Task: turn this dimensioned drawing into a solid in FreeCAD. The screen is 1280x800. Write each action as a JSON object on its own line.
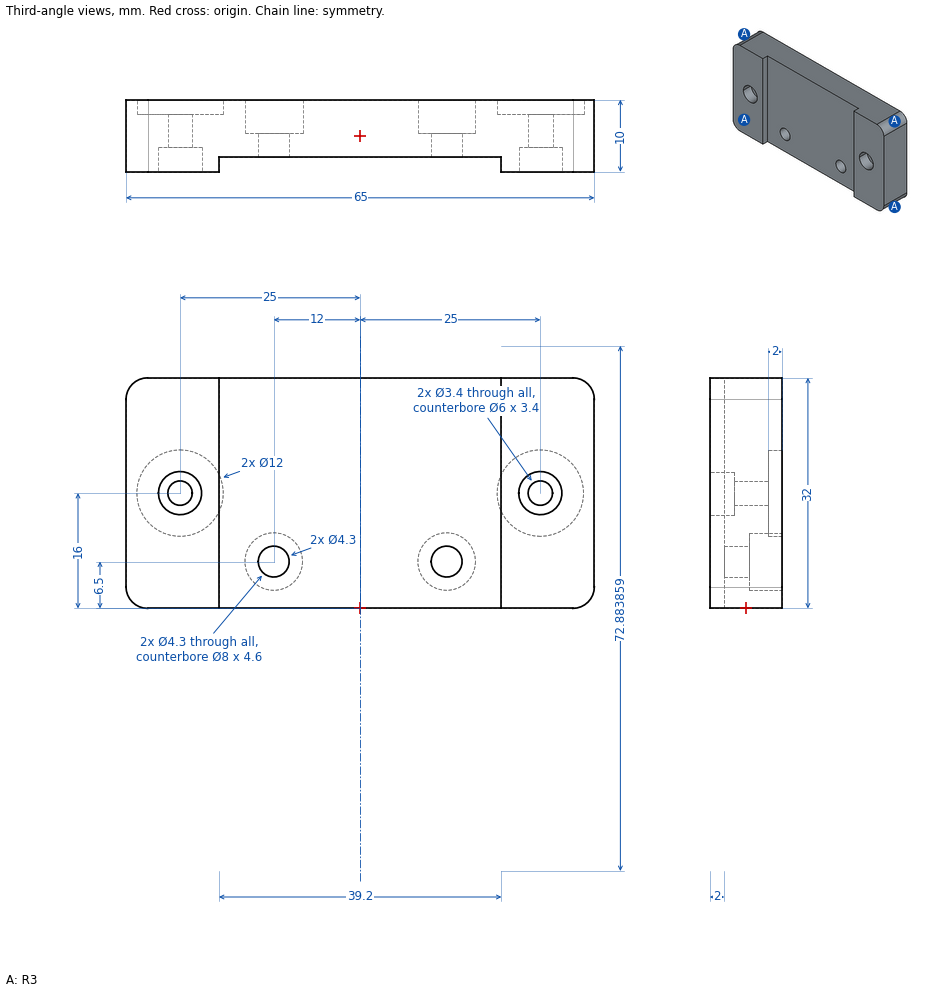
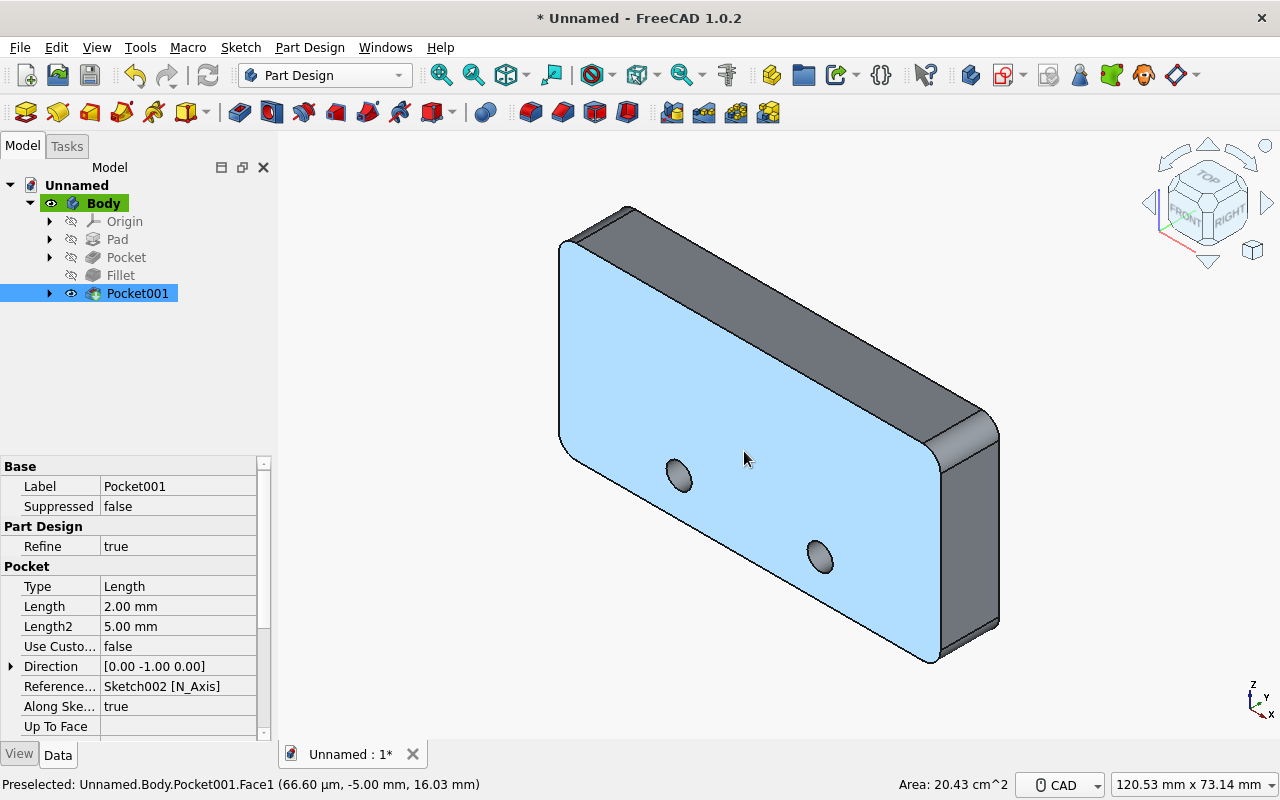
{"action": "left_click", "coordinate": [1004, 76]}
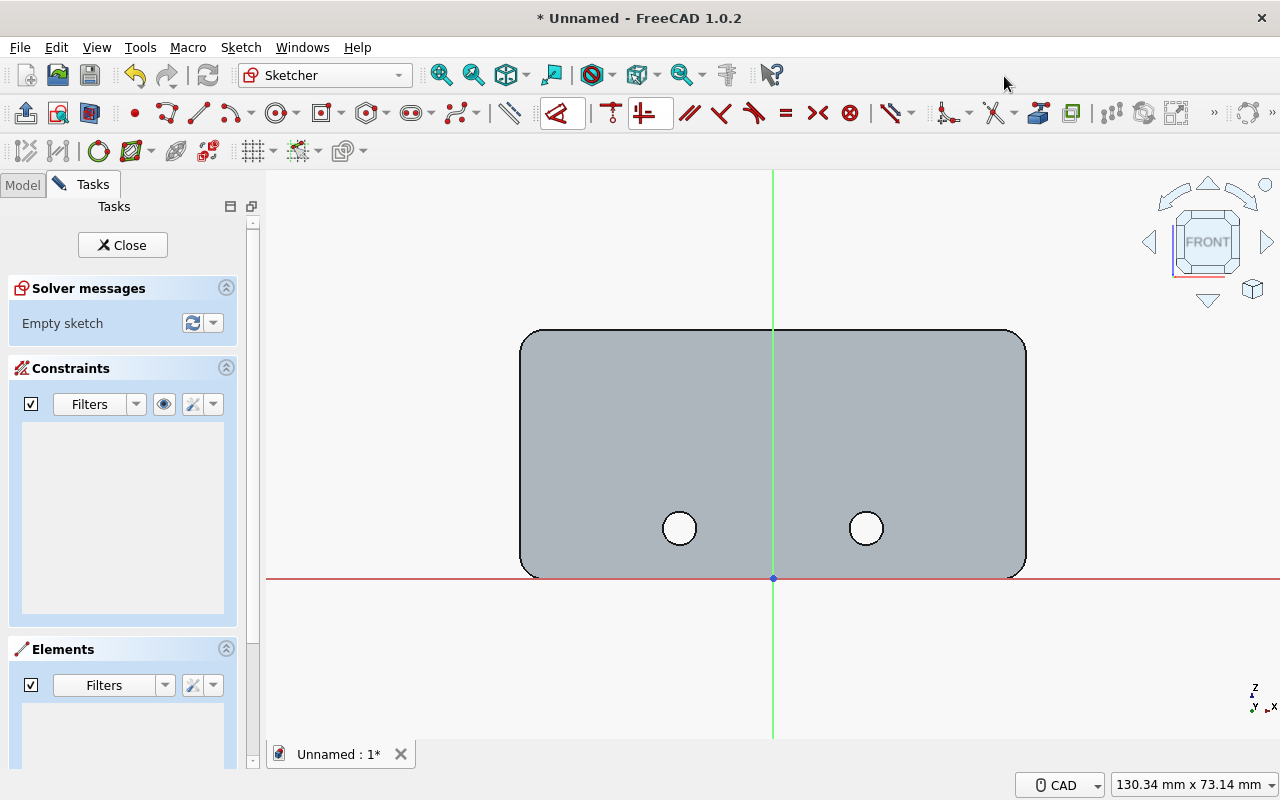
{"action": "scroll", "coordinate": [912, 623], "scroll_direction": "up", "scroll_amount": 2}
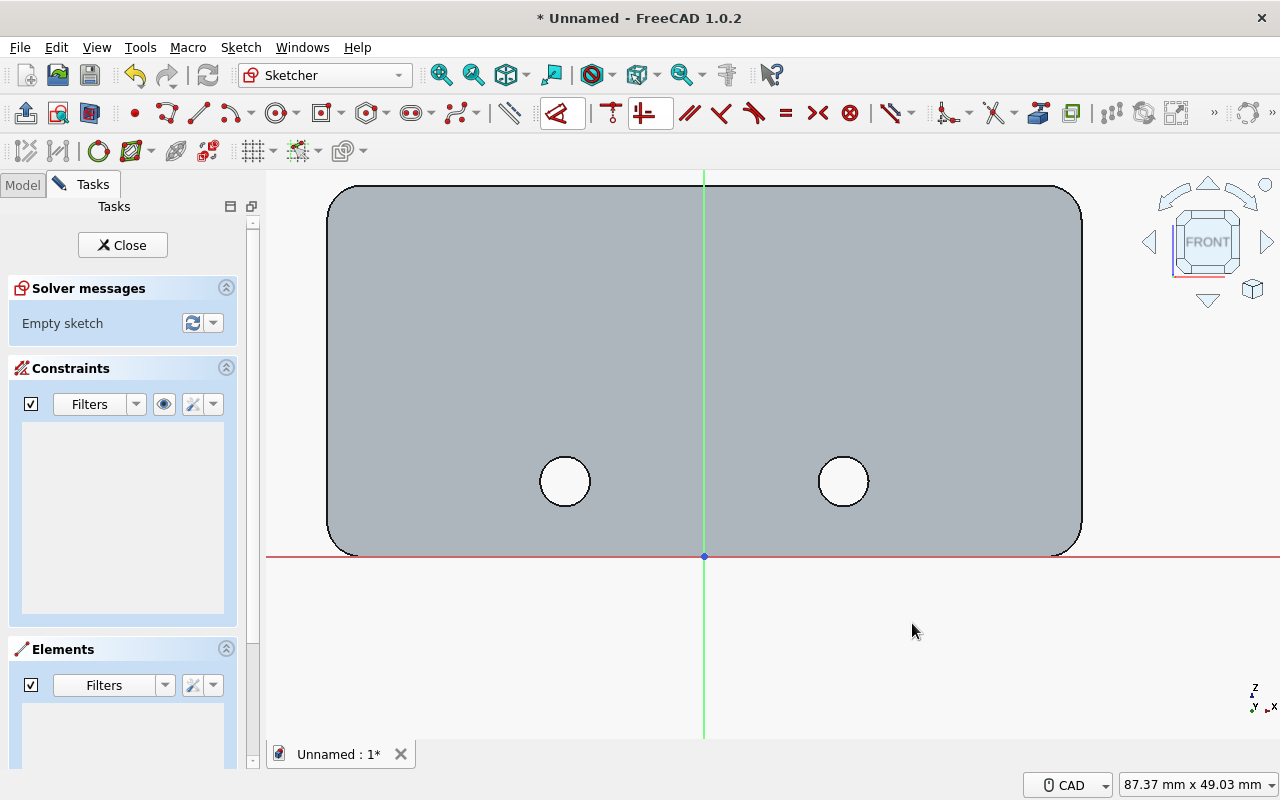
{"action": "left_click", "coordinate": [276, 114]}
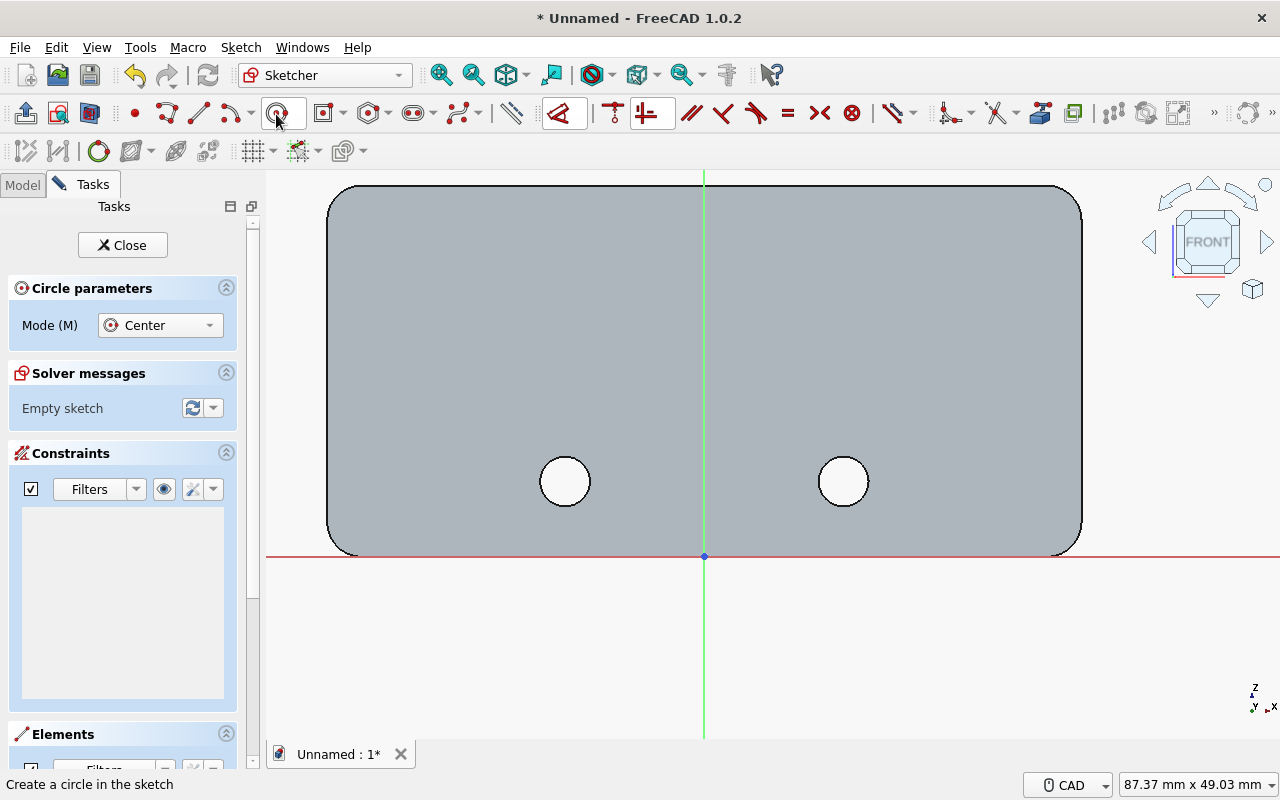
{"action": "left_click", "coordinate": [994, 371]}
{"action": "left_click", "coordinate": [1008, 357]}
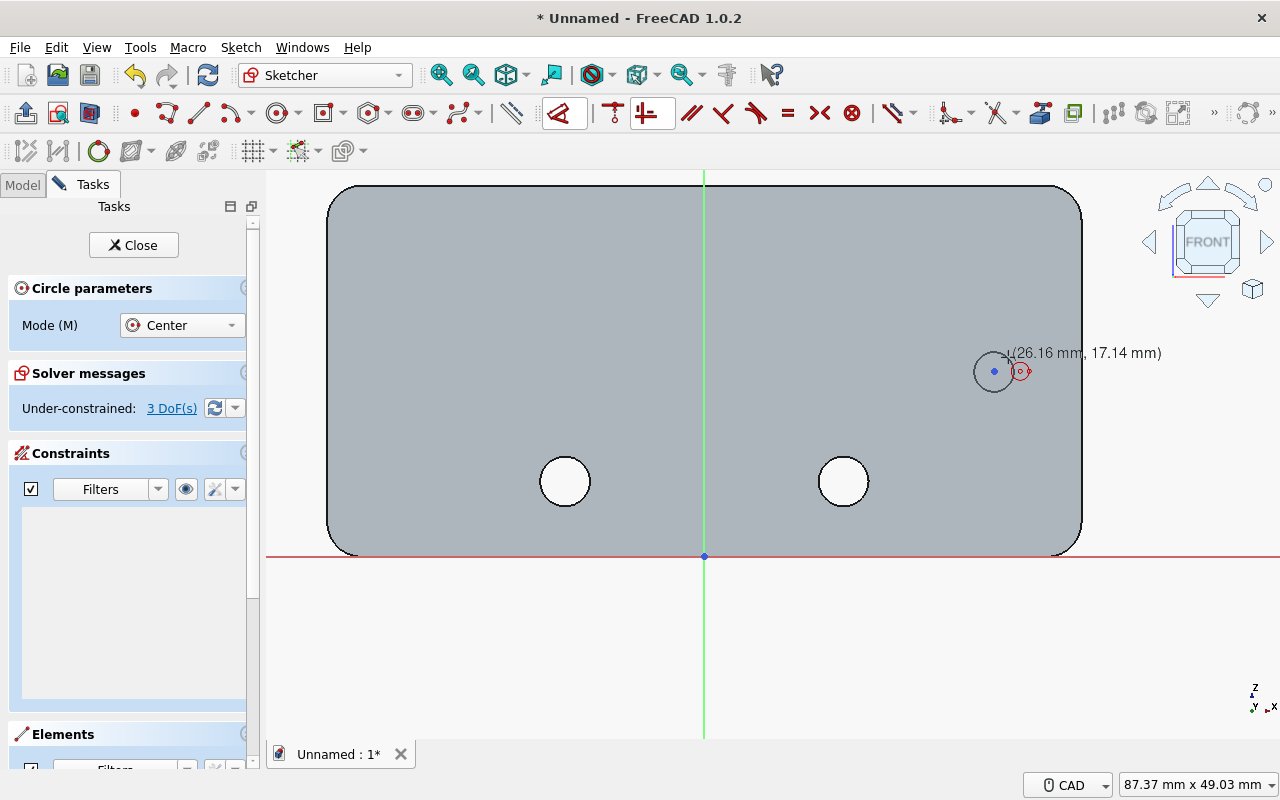
{"action": "left_click", "coordinate": [414, 371]}
{"action": "left_click", "coordinate": [428, 357]}
{"action": "key", "text": "Escape"}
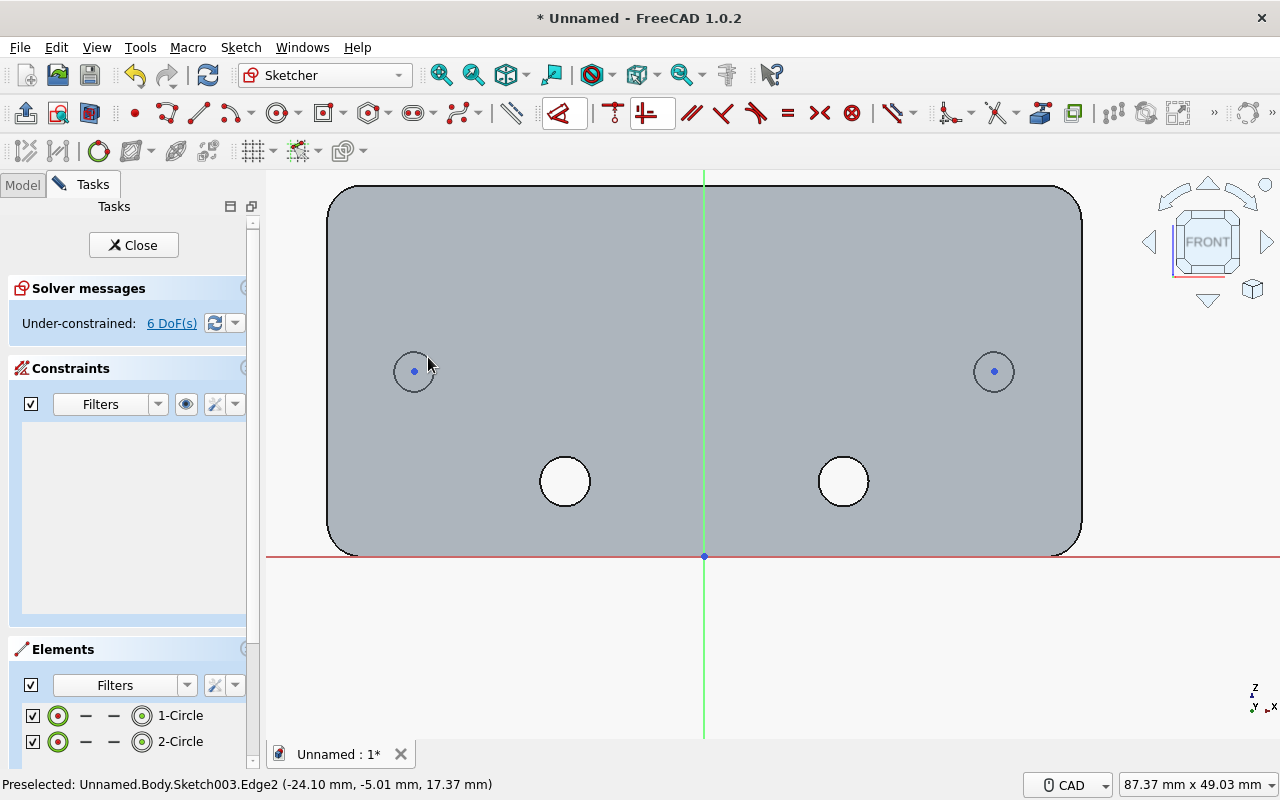
{"action": "left_click", "coordinate": [1008, 358]}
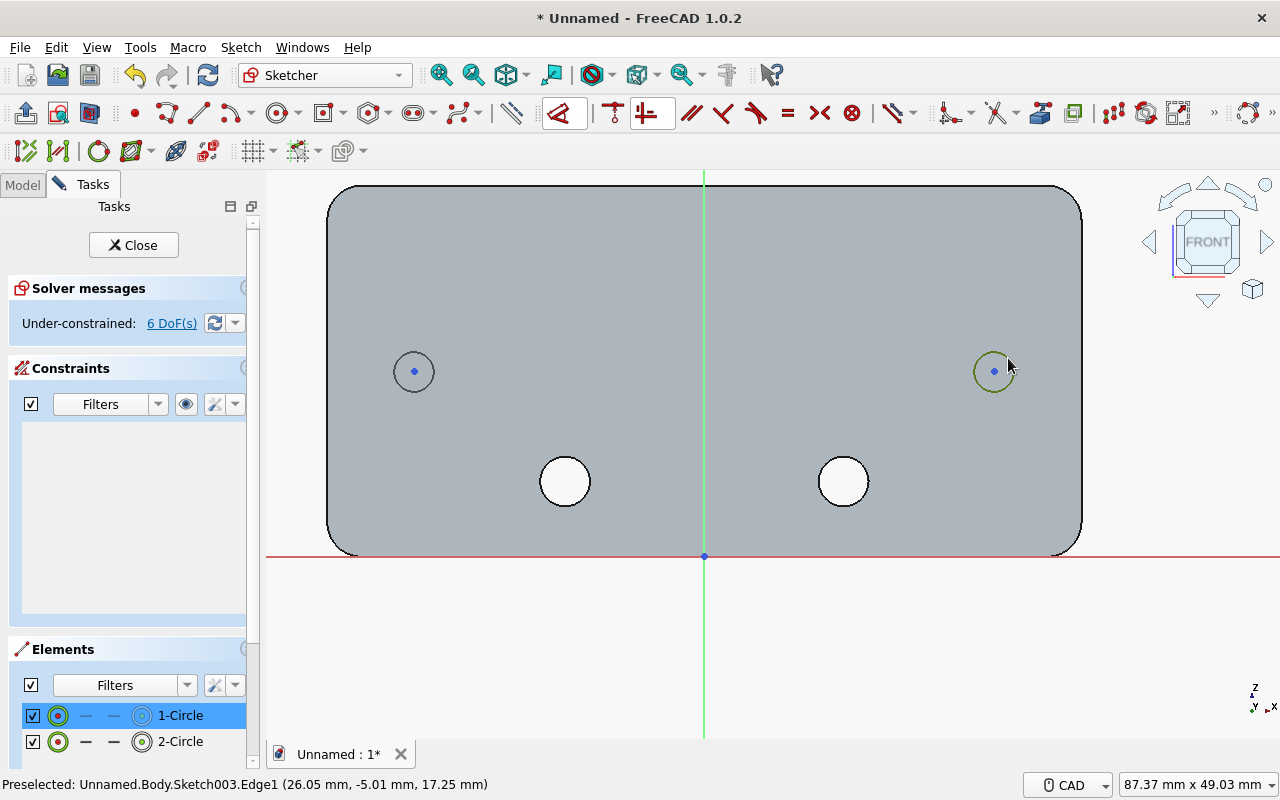
{"action": "left_click", "coordinate": [428, 358]}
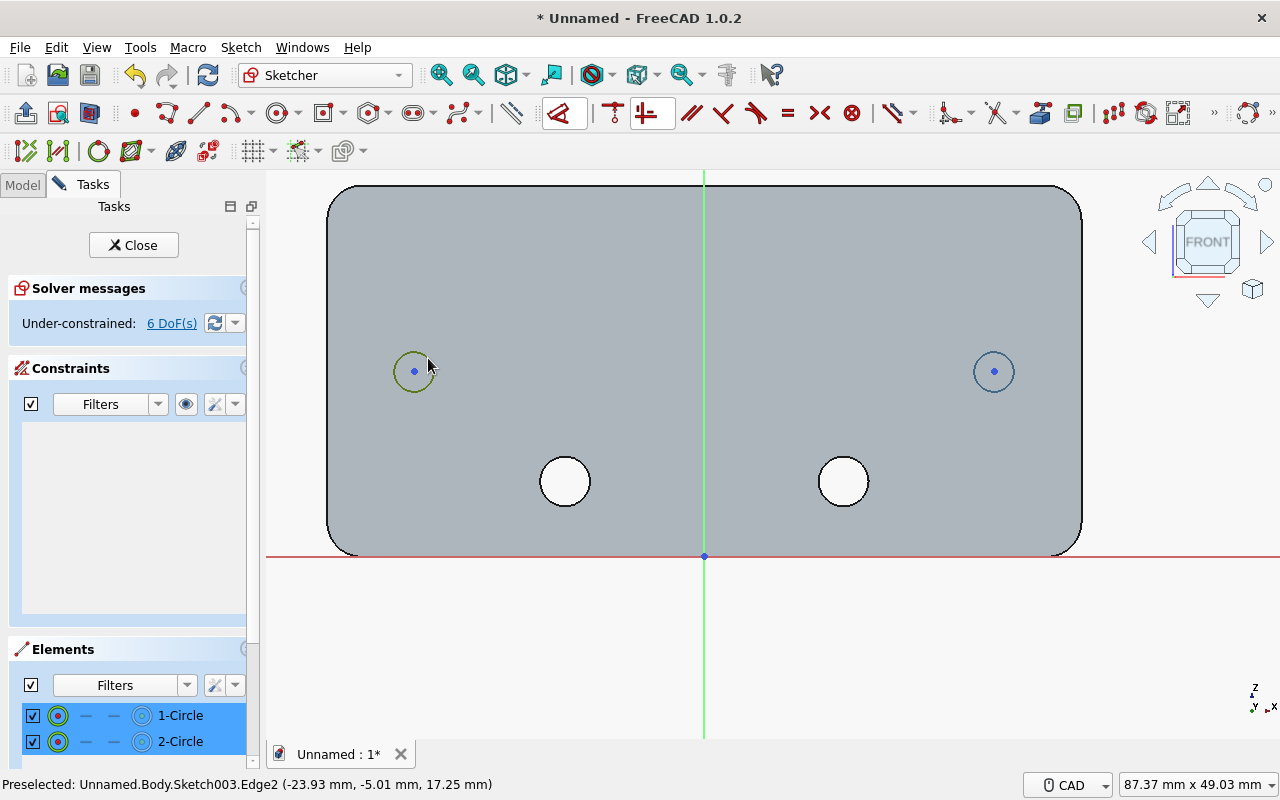
{"action": "left_click", "coordinate": [788, 114]}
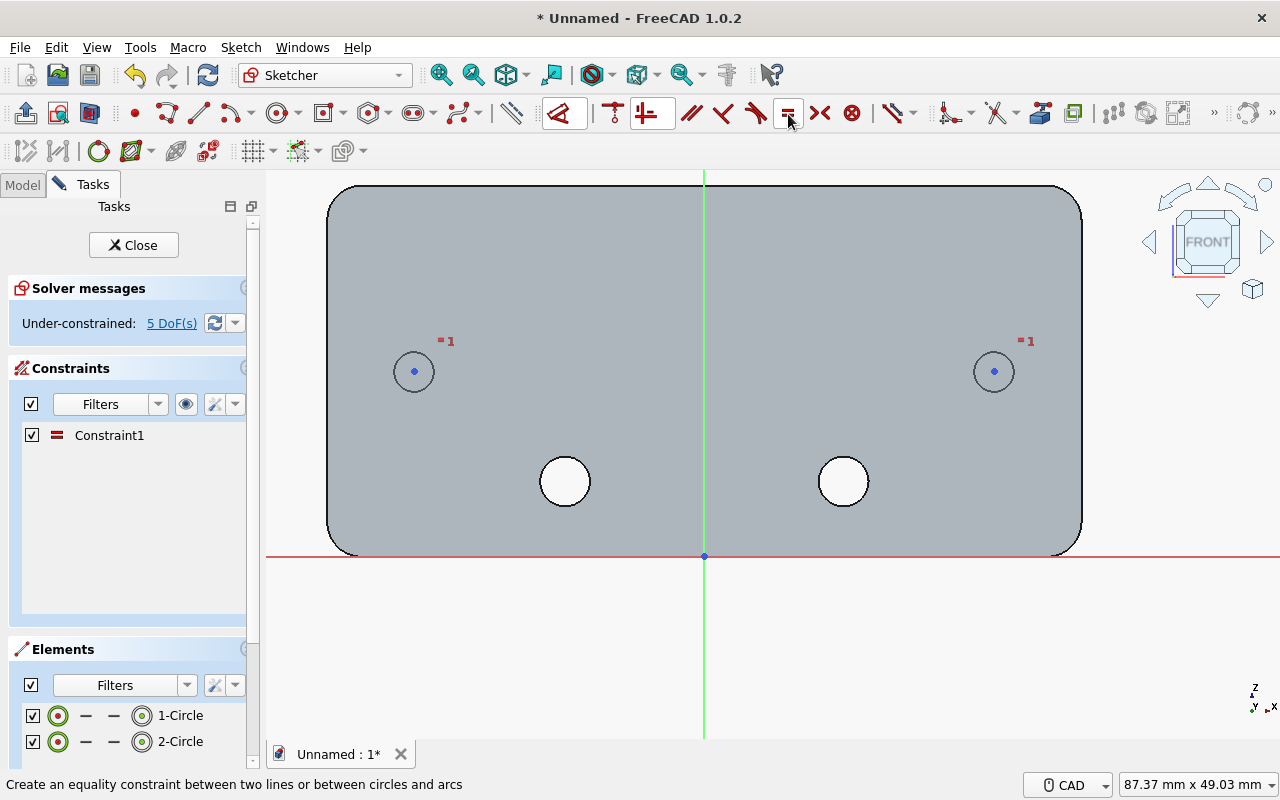
{"action": "left_click", "coordinate": [994, 372]}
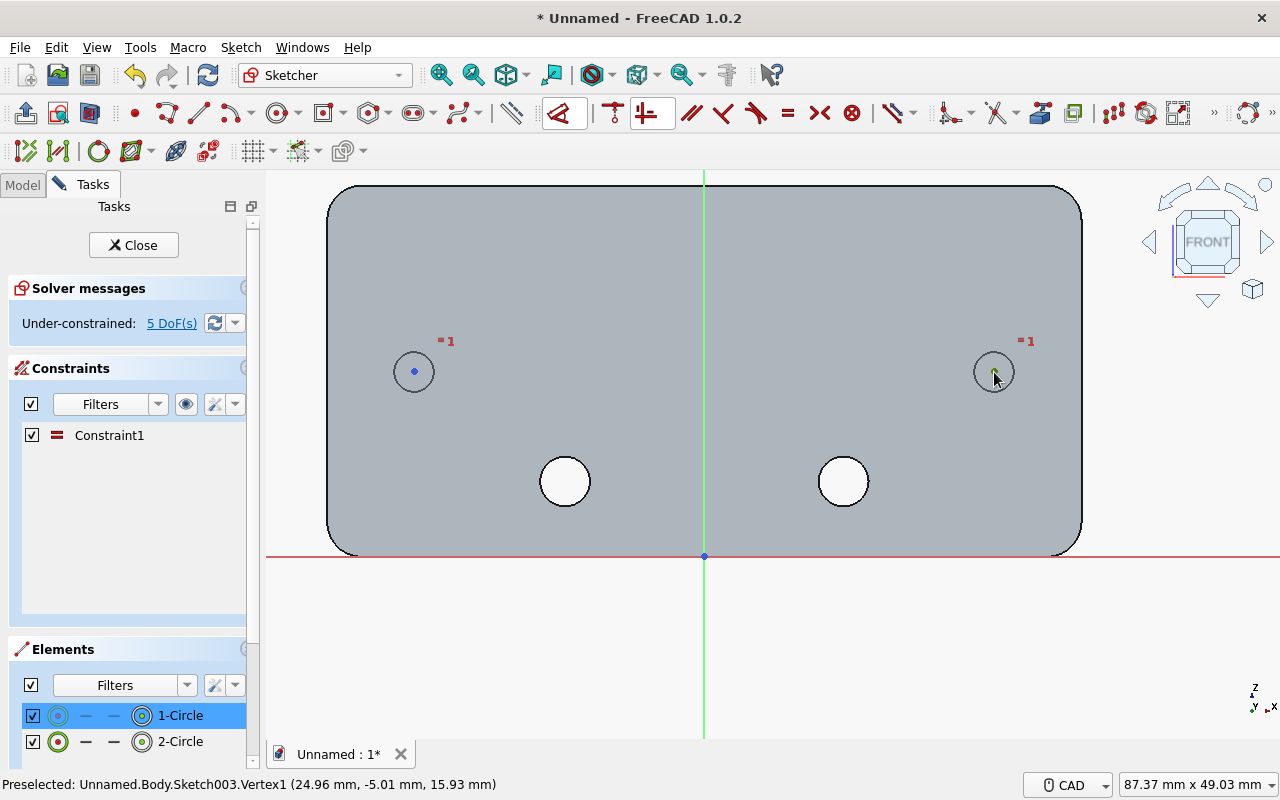
{"action": "left_click", "coordinate": [414, 372]}